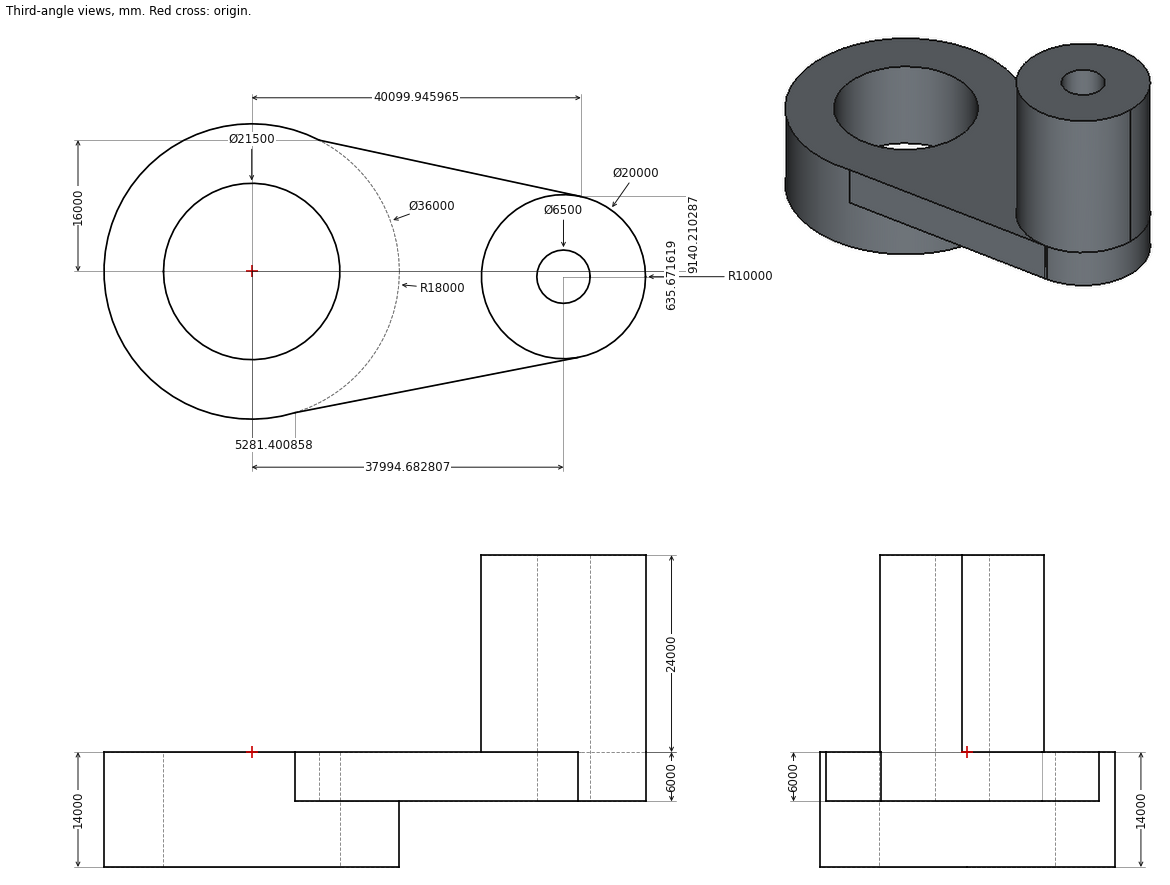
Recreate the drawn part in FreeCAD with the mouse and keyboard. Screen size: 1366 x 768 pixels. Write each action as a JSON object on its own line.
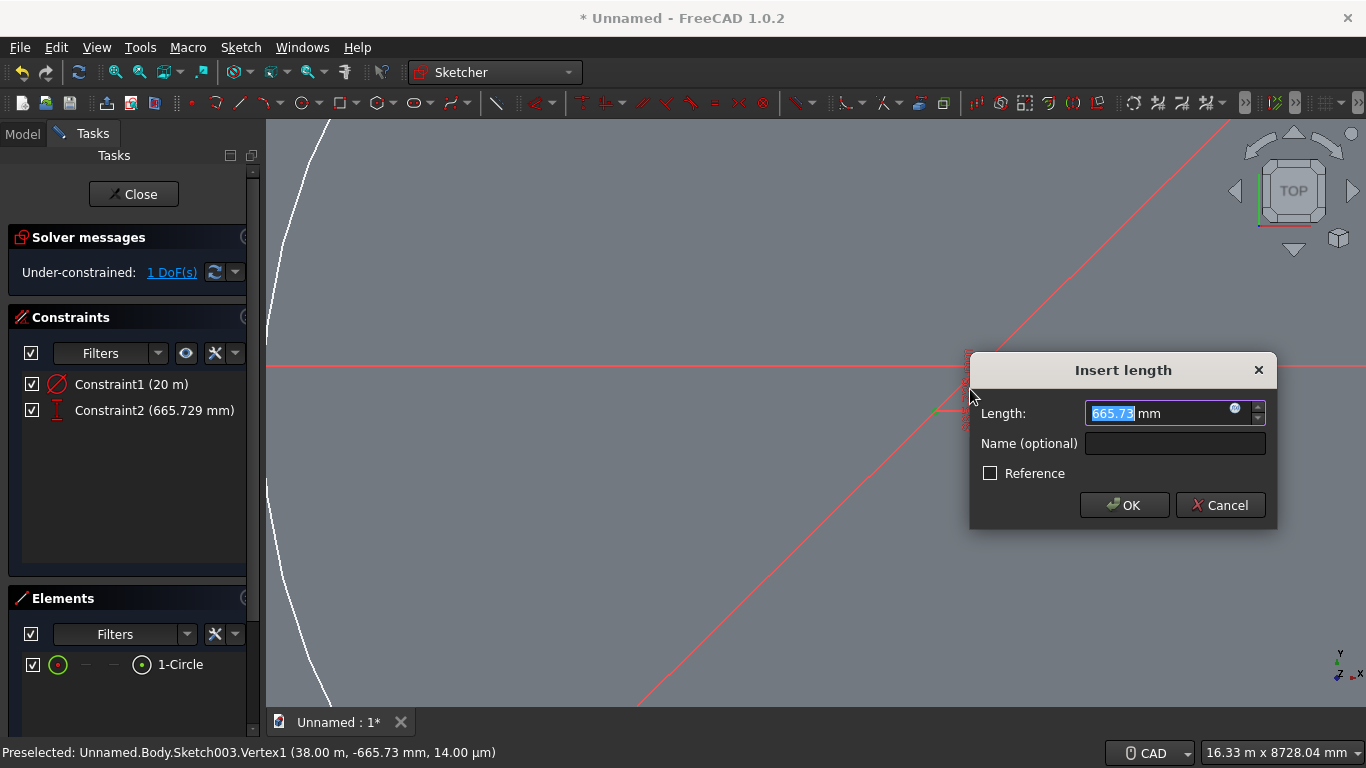
{"action": "type", "text": "635.671619"}
{"action": "key", "text": "Return"}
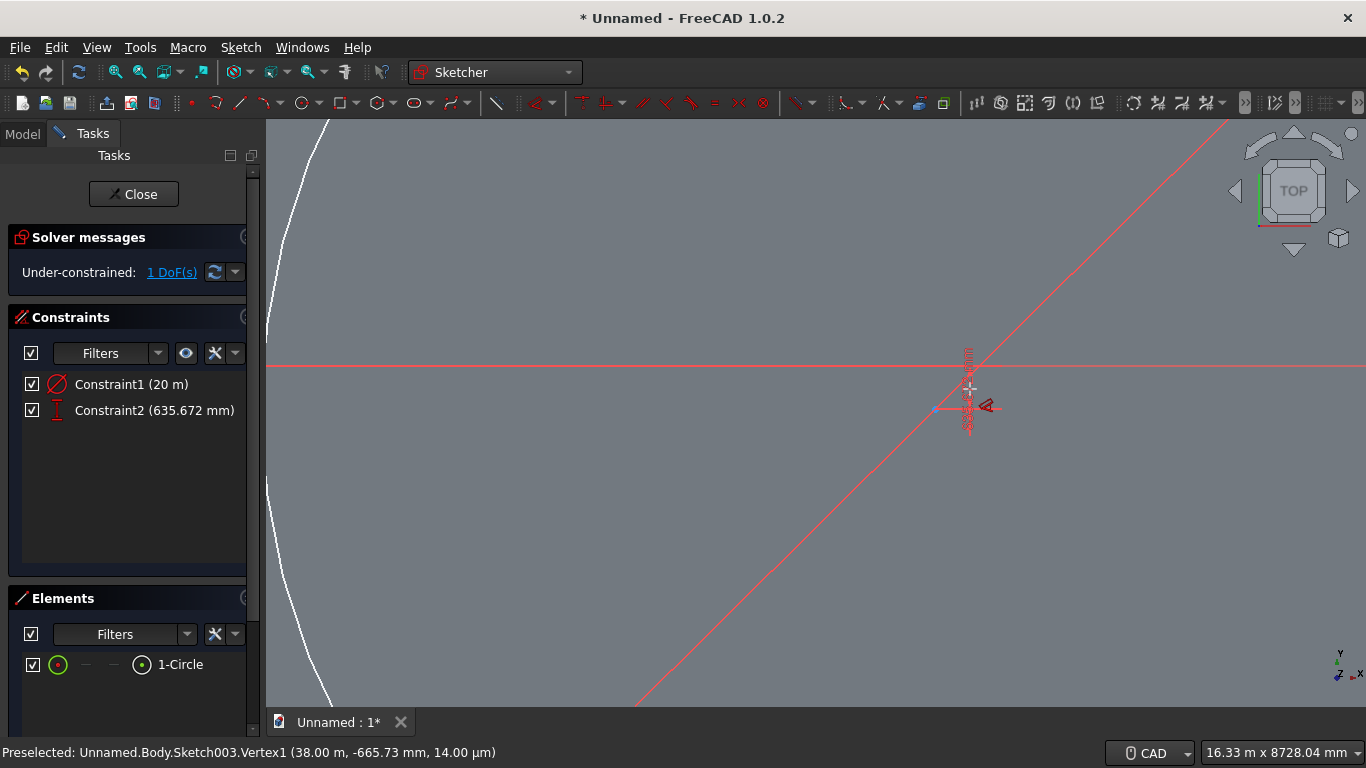
{"action": "scroll", "coordinate": [939, 414], "scroll_direction": "down", "scroll_amount": 8}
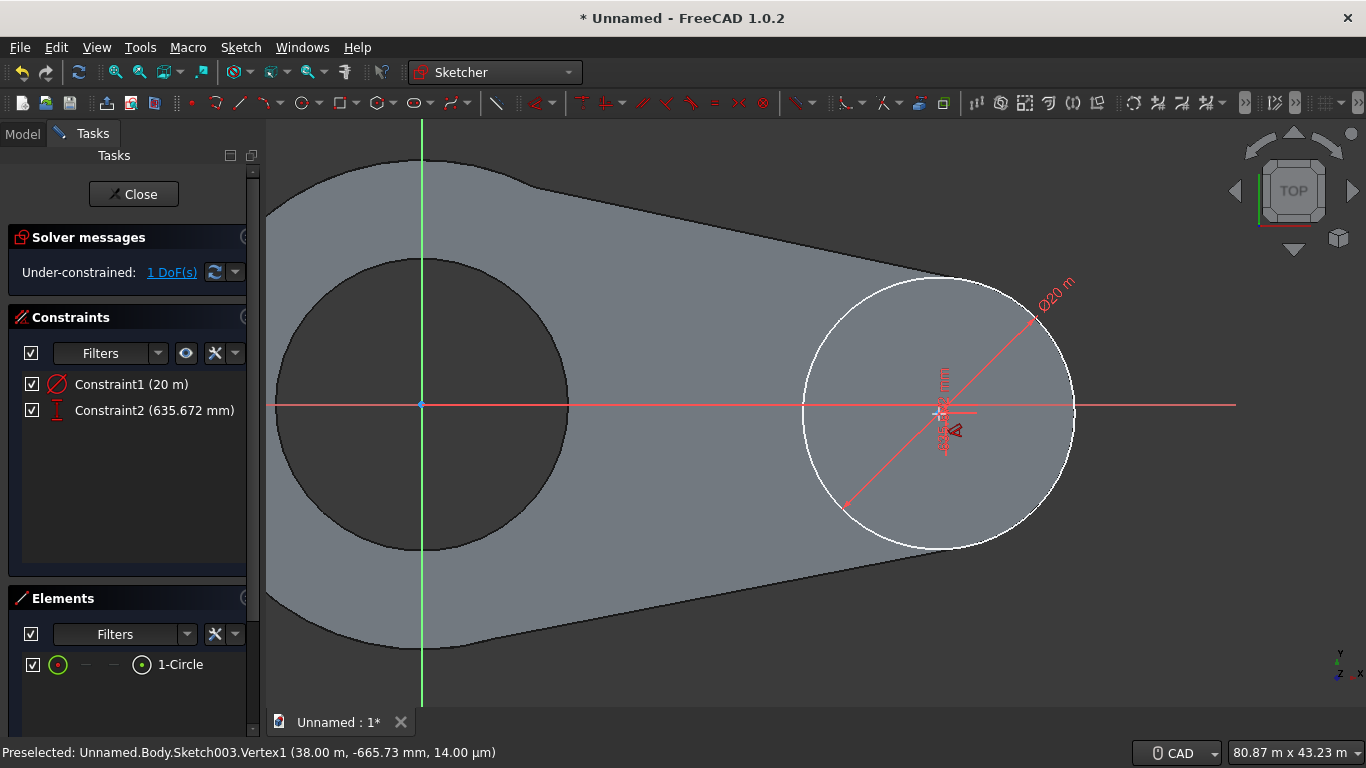
{"action": "left_click", "coordinate": [939, 413]}
{"action": "left_click", "coordinate": [680, 371]}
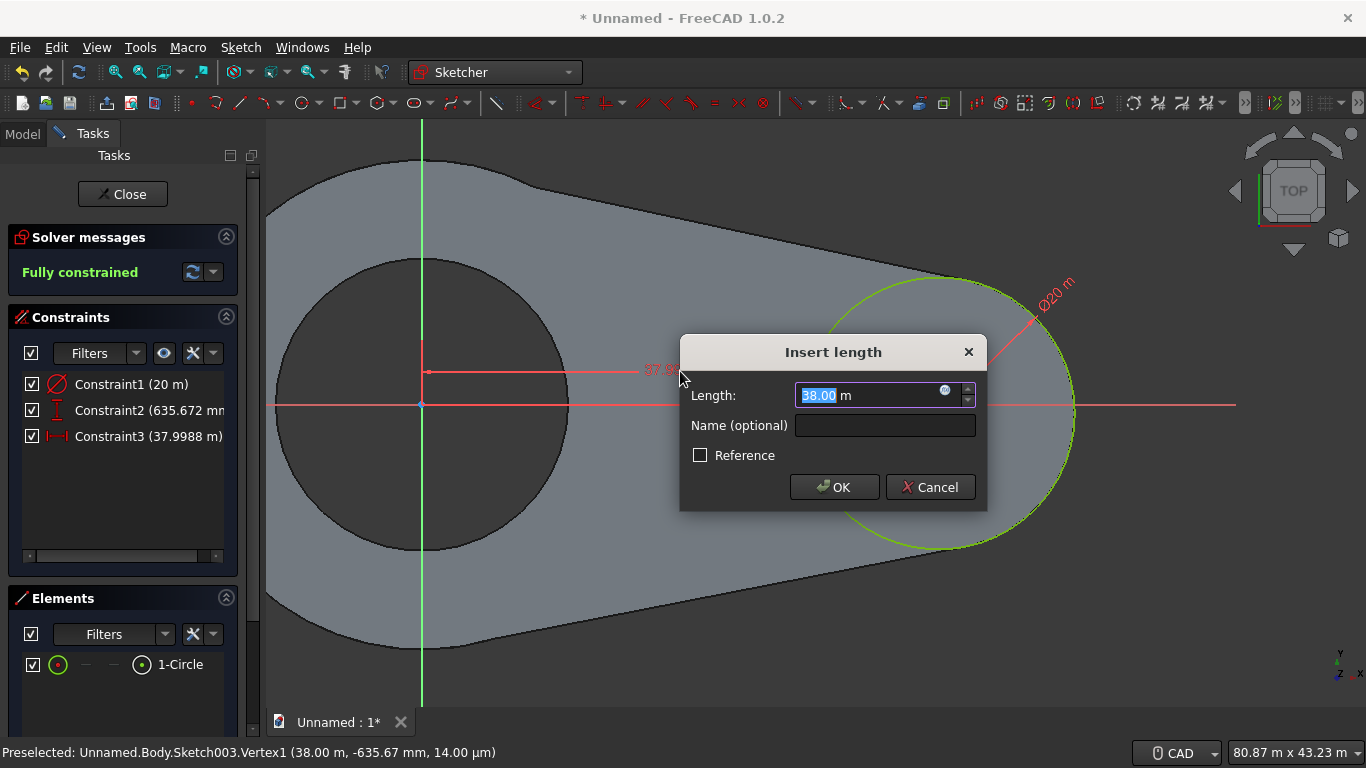
{"action": "key", "text": "ctrl+a"}
{"action": "type", "text": "37994.682807 mm"}
{"action": "key", "text": "Return"}
{"action": "key", "text": "Escape"}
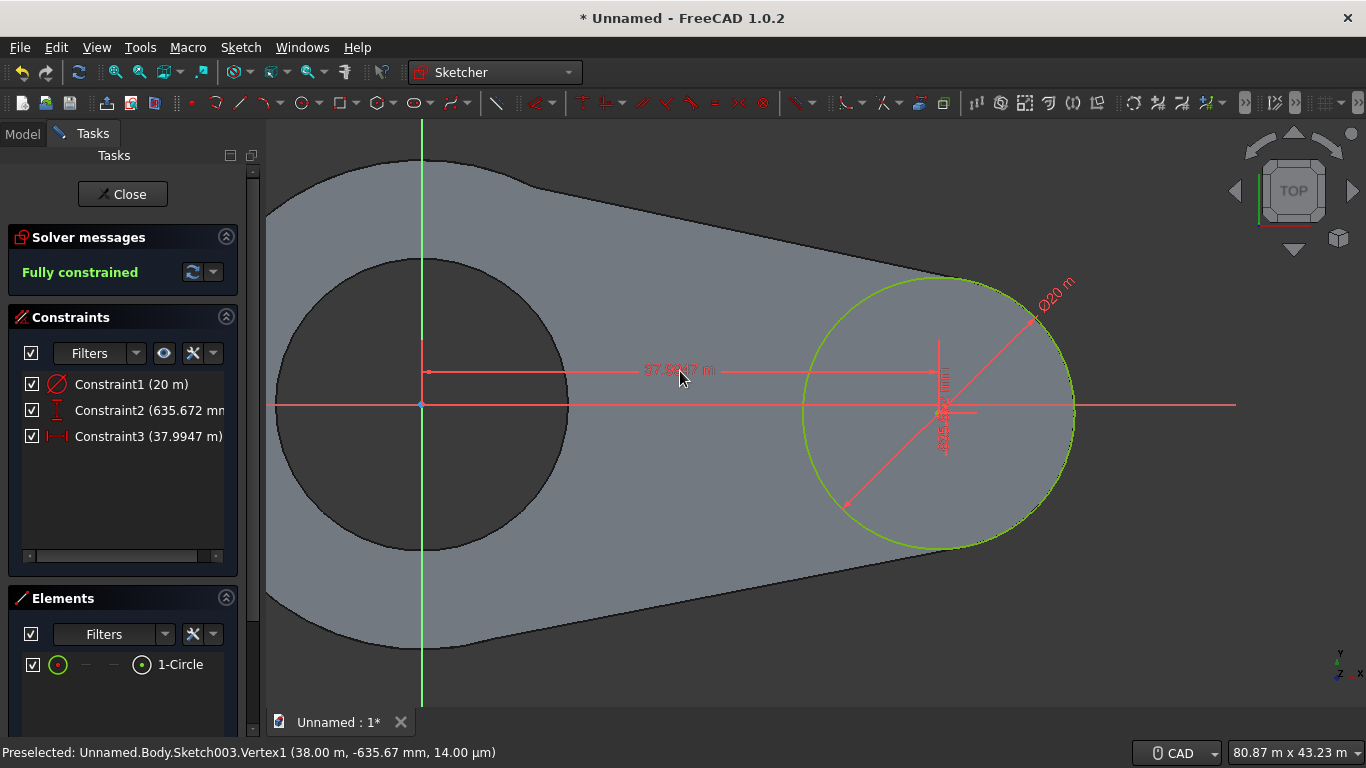
{"action": "left_click", "coordinate": [123, 194]}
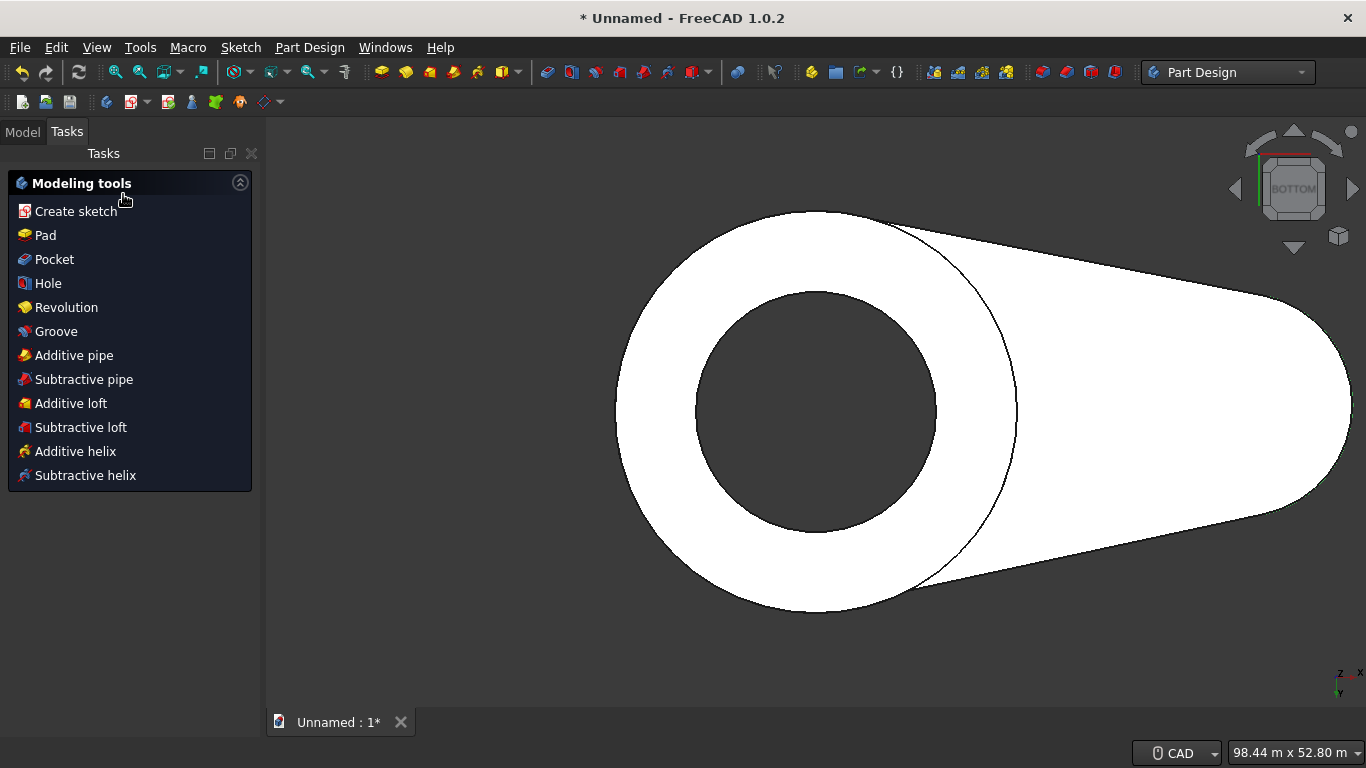
{"action": "left_click", "coordinate": [382, 72]}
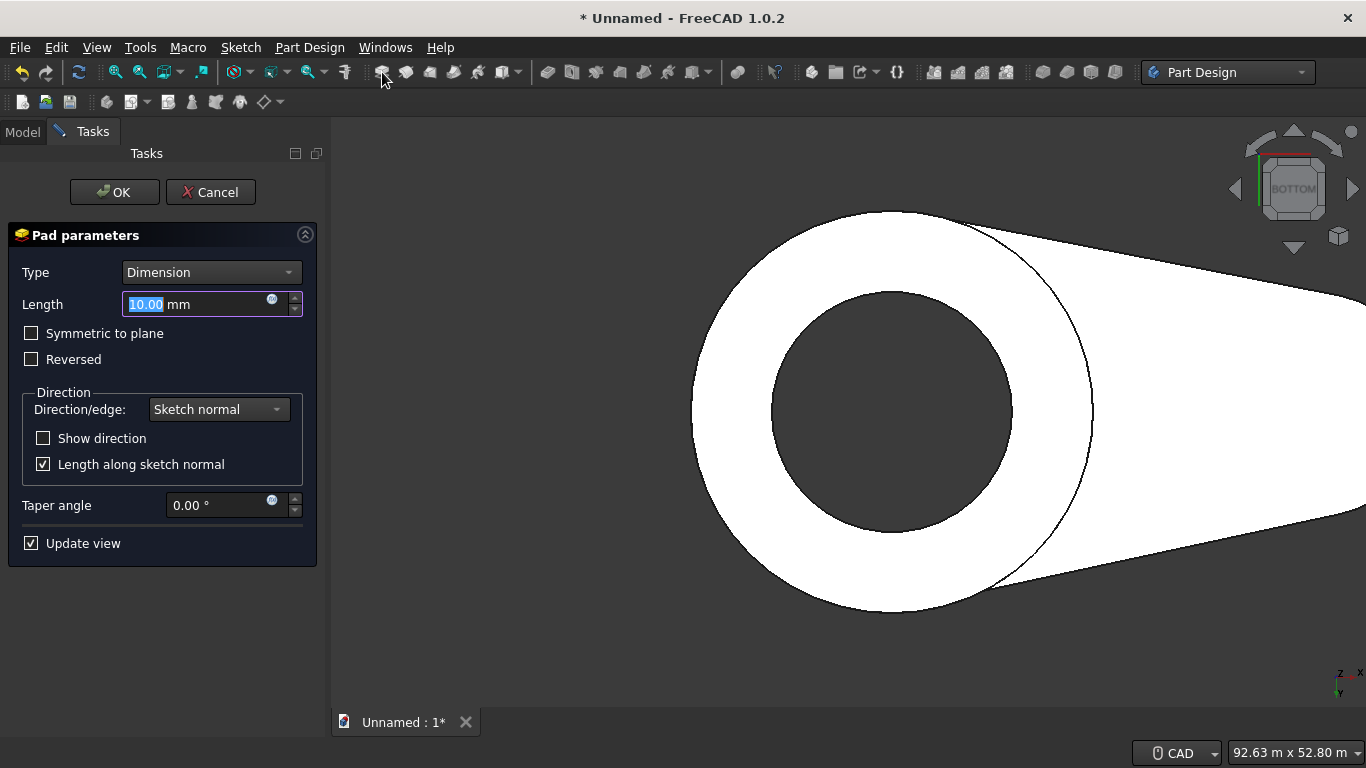
{"action": "left_click", "coordinate": [212, 272]}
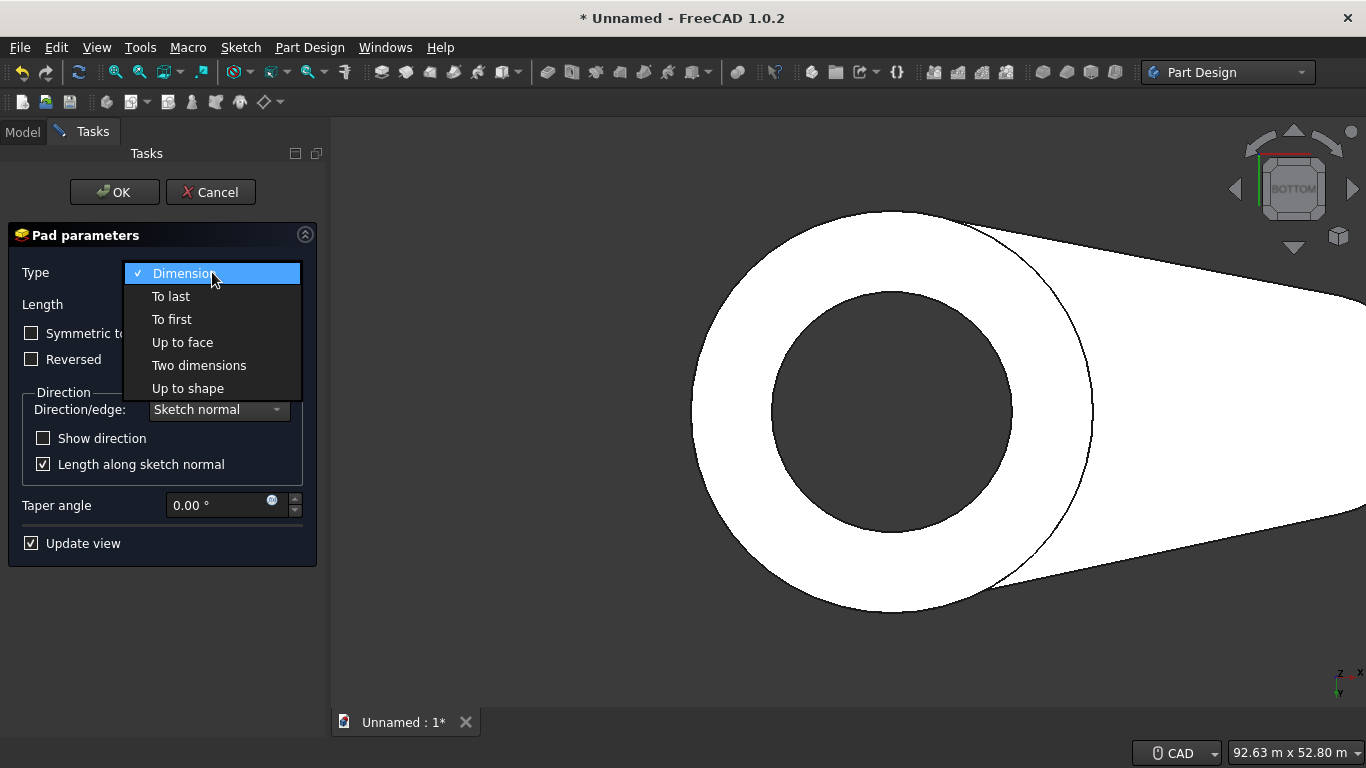
{"action": "left_click", "coordinate": [212, 366]}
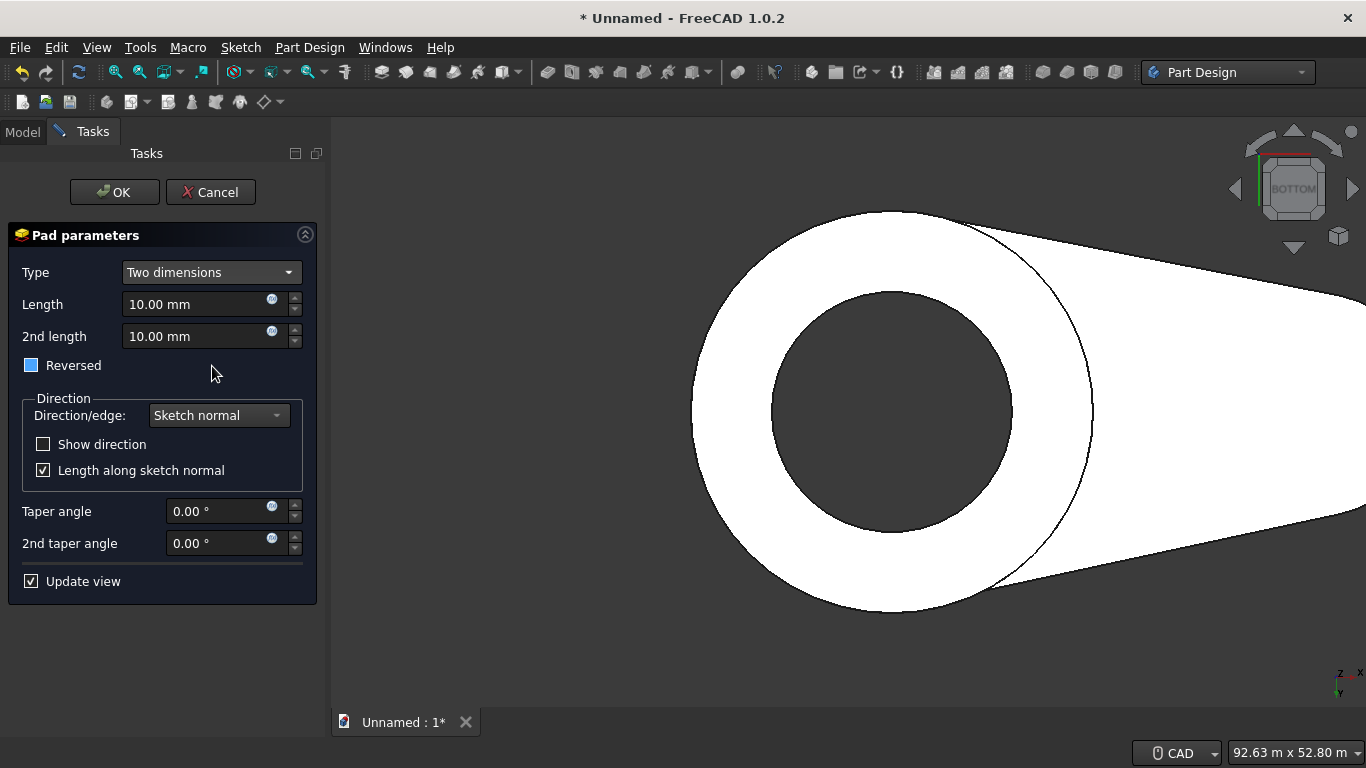
{"action": "triple_click", "coordinate": [204, 304]}